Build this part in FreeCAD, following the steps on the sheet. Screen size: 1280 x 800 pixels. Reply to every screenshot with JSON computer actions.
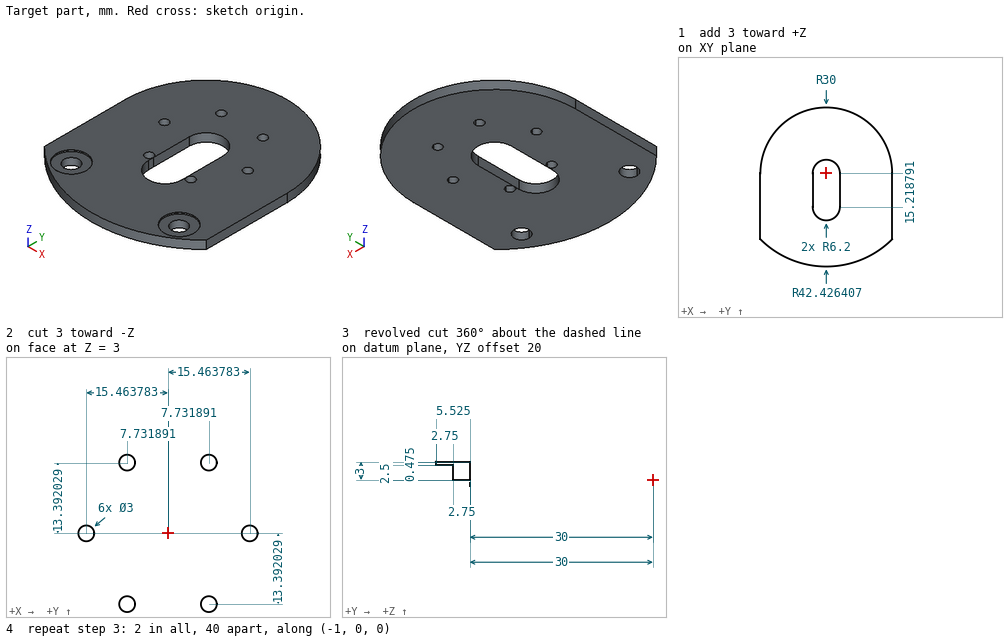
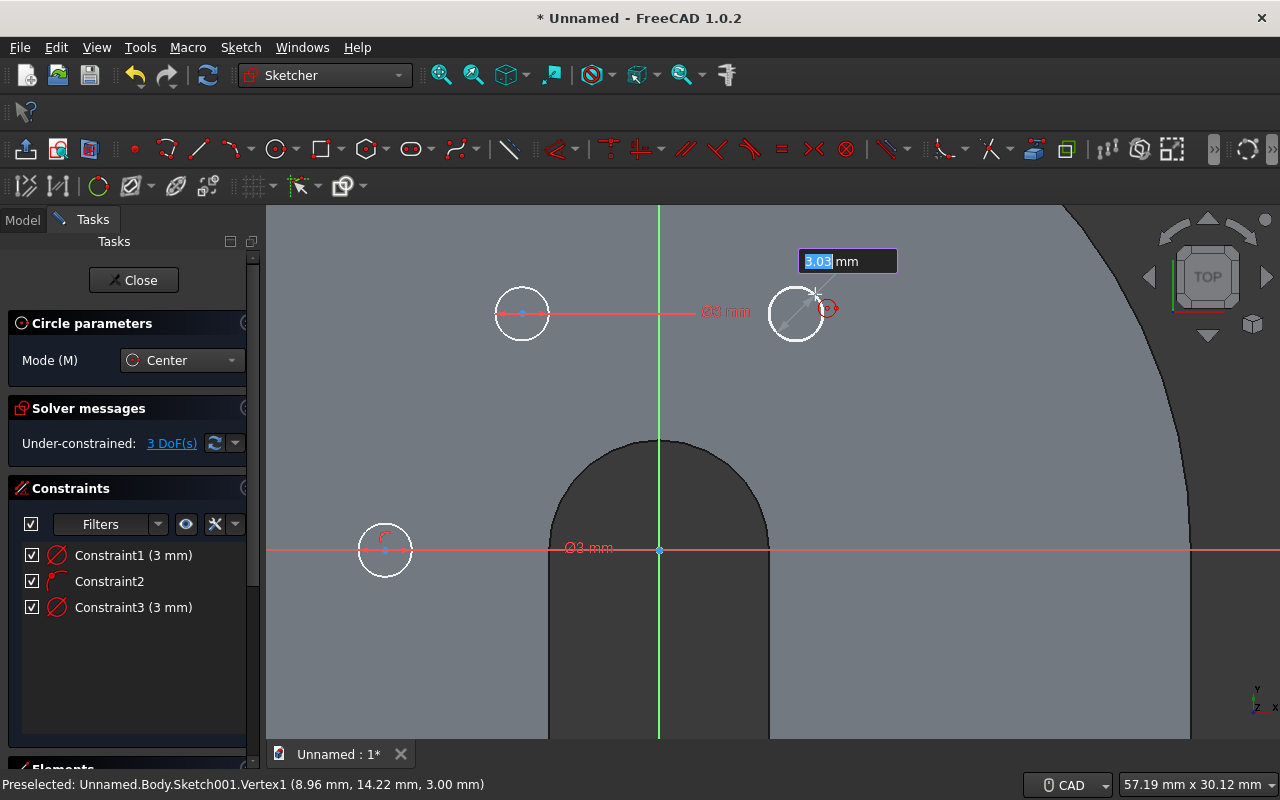
{"action": "type", "text": "3"}
{"action": "key", "text": "Return"}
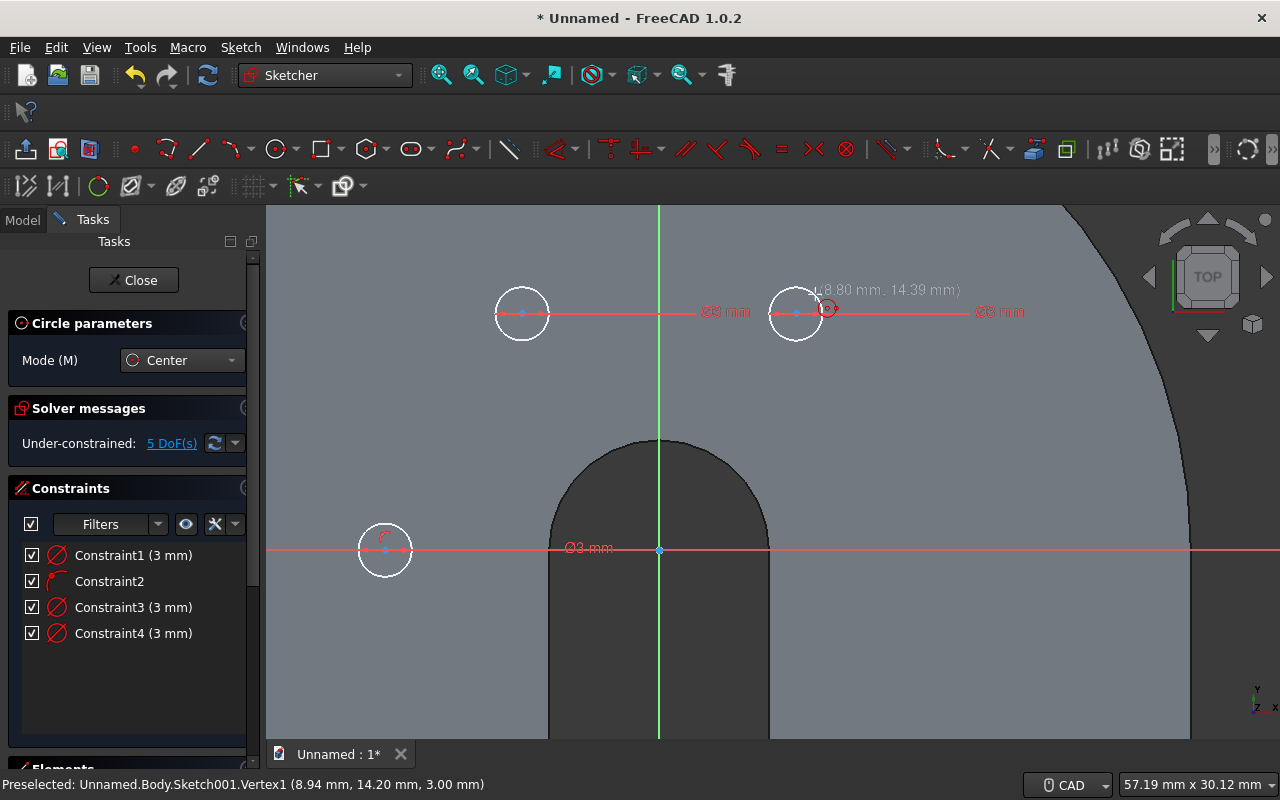
{"action": "left_click", "coordinate": [933, 550]}
{"action": "mouse_move", "coordinate": [952, 531]}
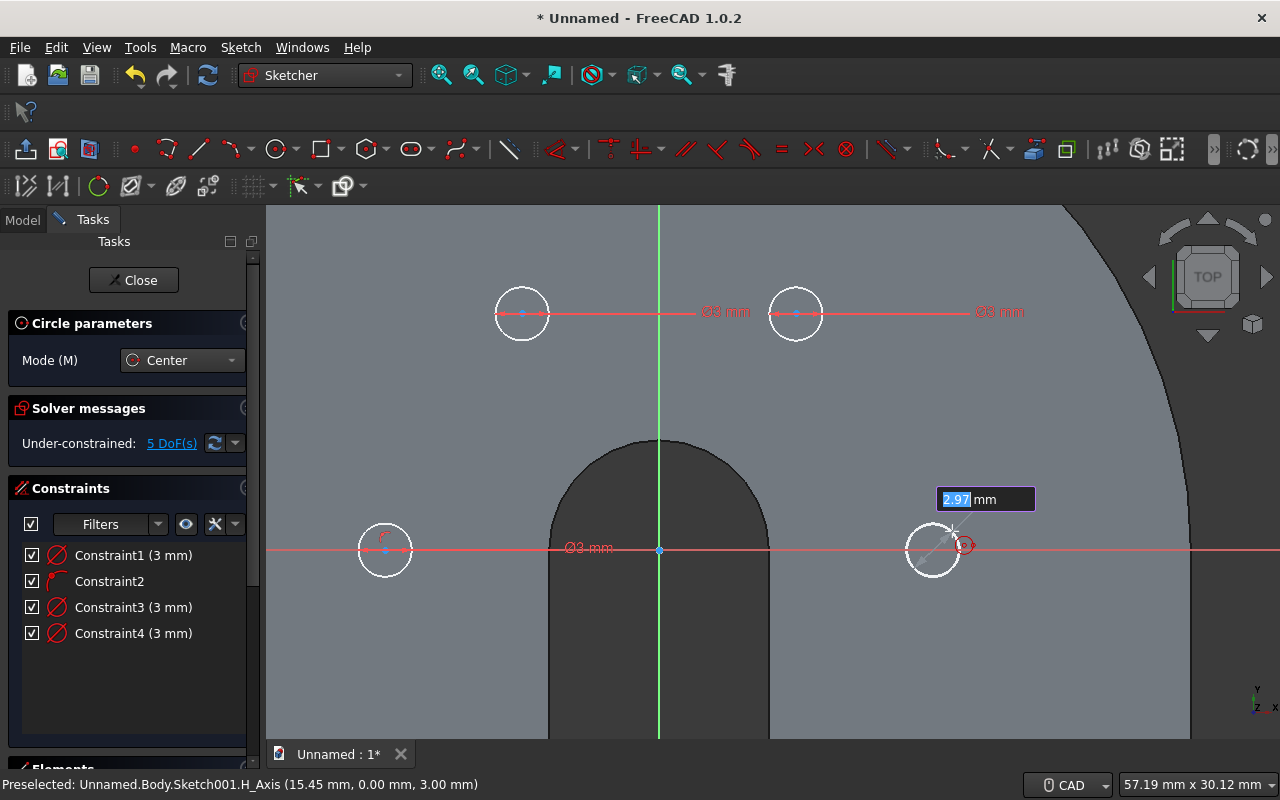
{"action": "type", "text": "3"}
{"action": "key", "text": "Return"}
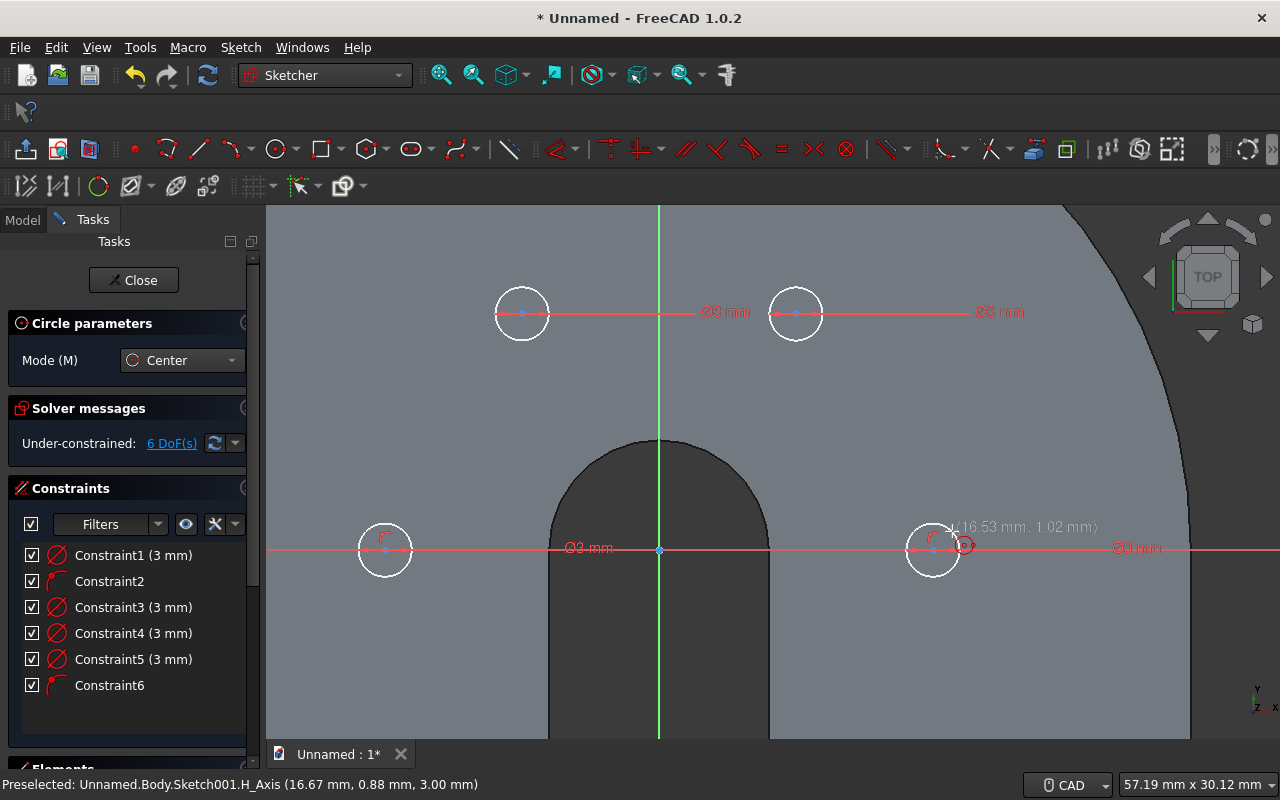
{"action": "scroll", "coordinate": [797, 313], "scroll_direction": "down", "scroll_amount": 2}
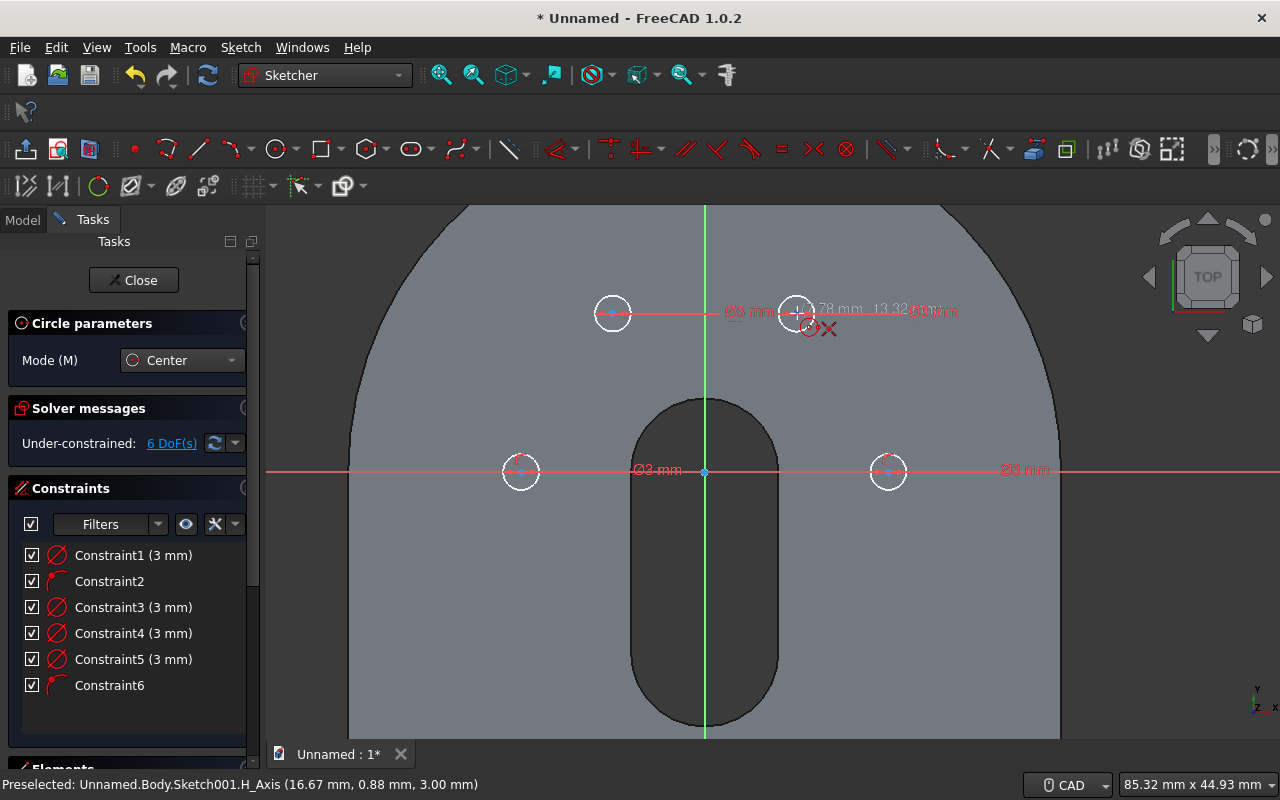
{"action": "scroll", "coordinate": [797, 631], "scroll_direction": "up", "scroll_amount": 2}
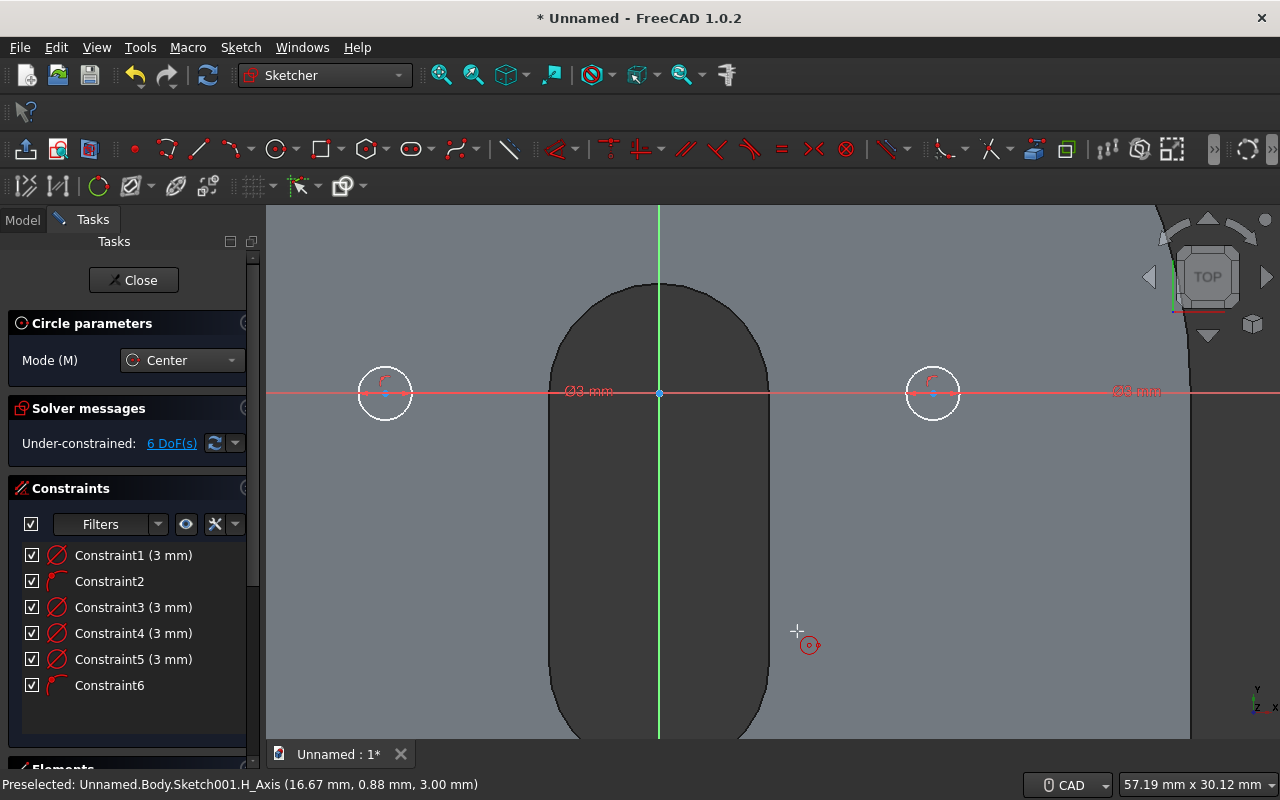
{"action": "left_click", "coordinate": [796, 631]}
{"action": "mouse_move", "coordinate": [815, 612]}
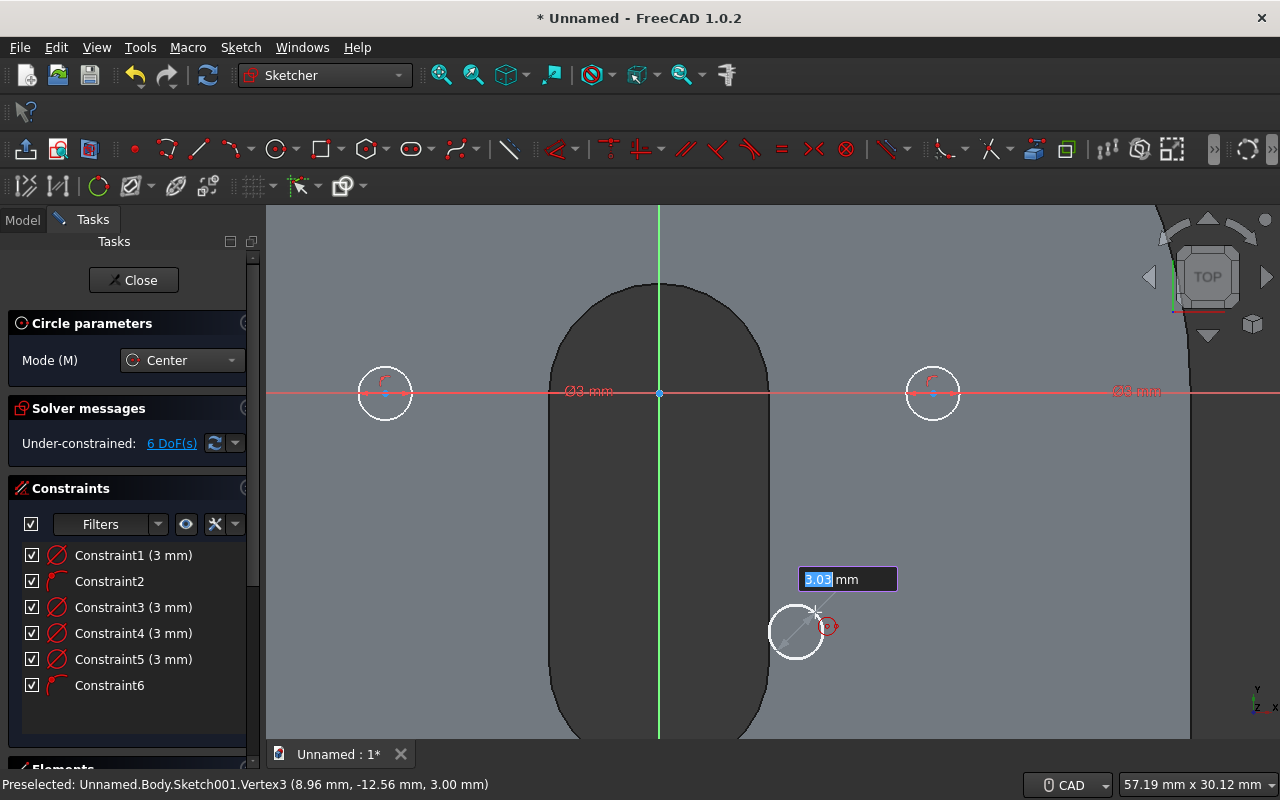
{"action": "type", "text": "3"}
{"action": "key", "text": "Return"}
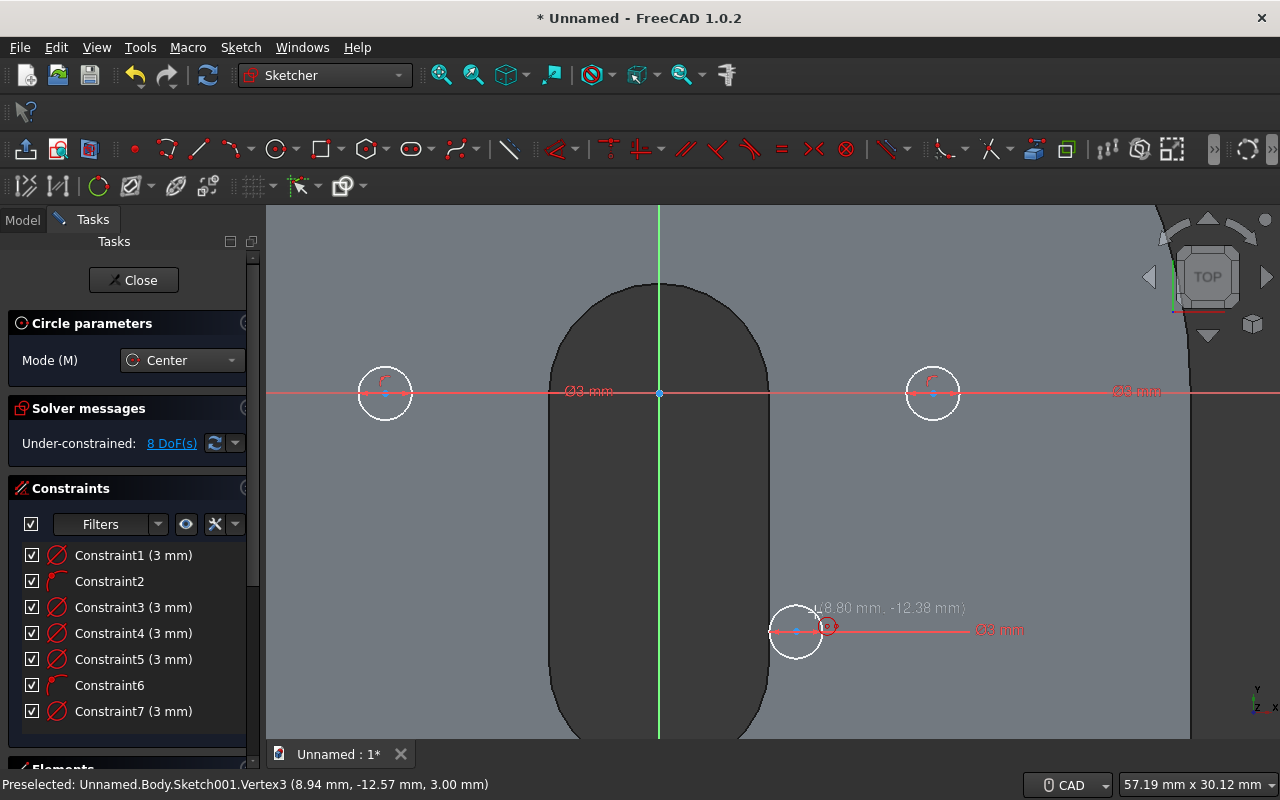
{"action": "left_click", "coordinate": [522, 631]}
{"action": "mouse_move", "coordinate": [541, 612]}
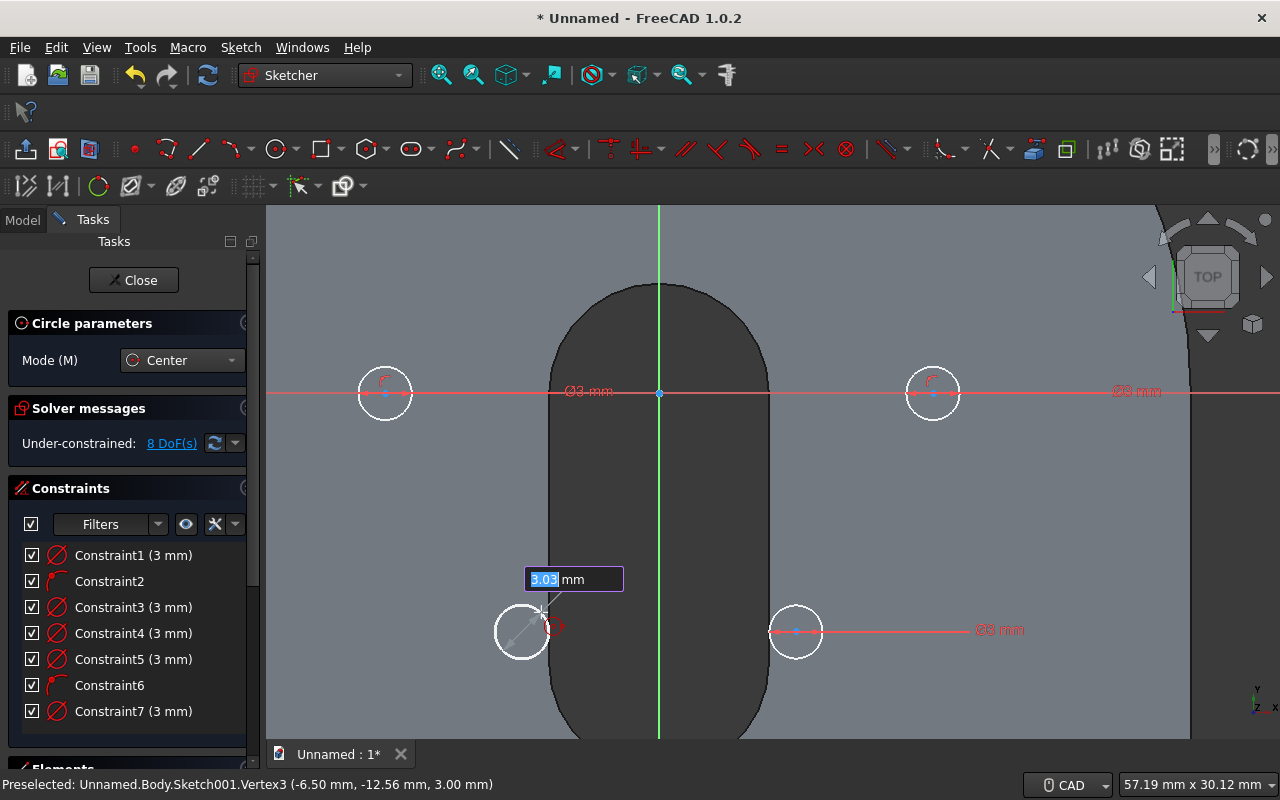
{"action": "type", "text": "3"}
{"action": "key", "text": "Return"}
{"action": "key", "text": "Escape"}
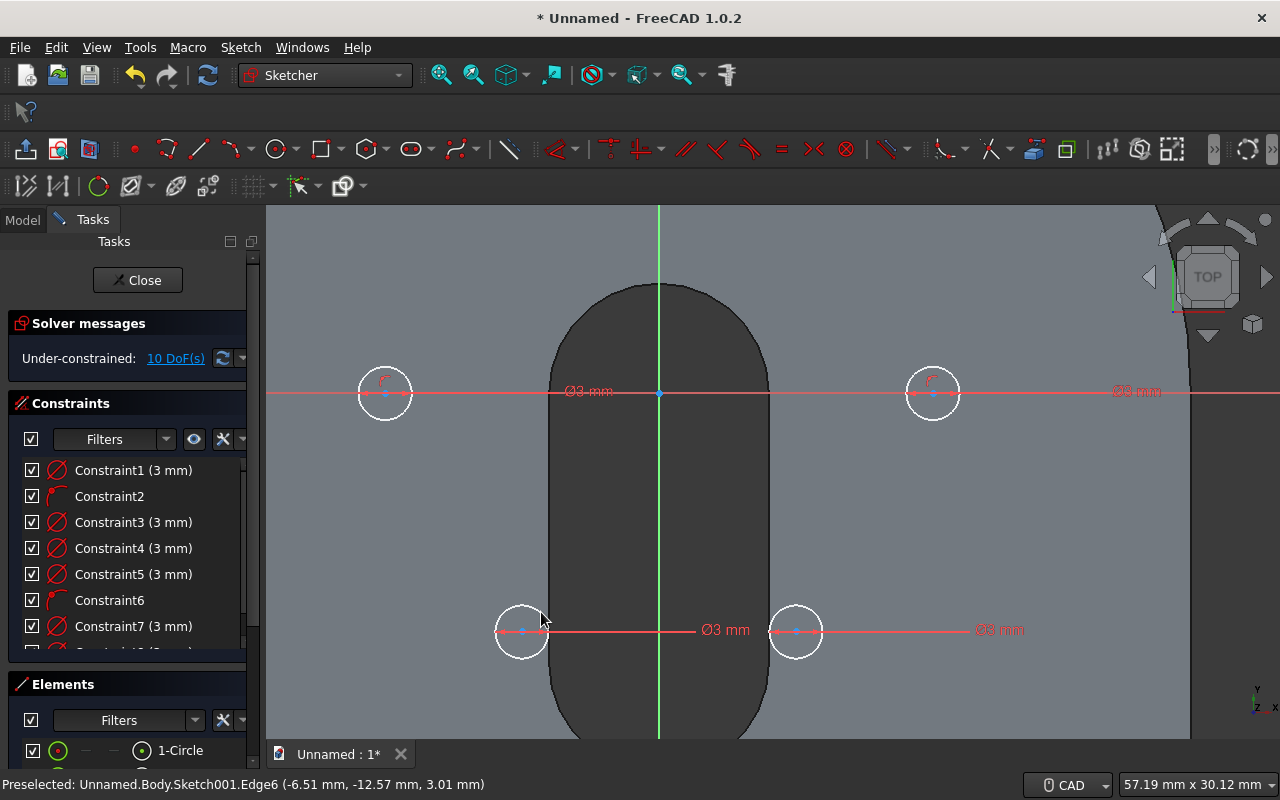
{"action": "scroll", "coordinate": [797, 632], "scroll_direction": "down", "scroll_amount": 2}